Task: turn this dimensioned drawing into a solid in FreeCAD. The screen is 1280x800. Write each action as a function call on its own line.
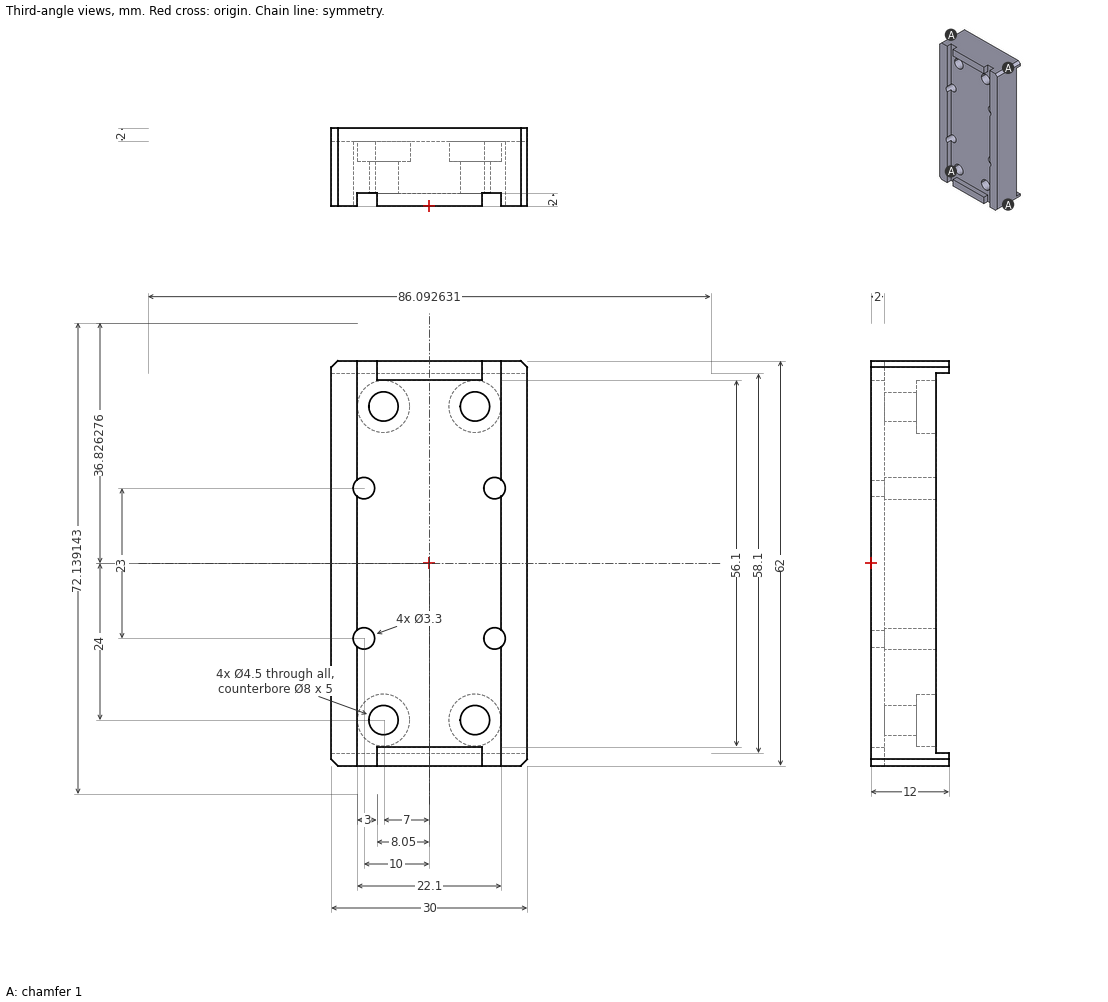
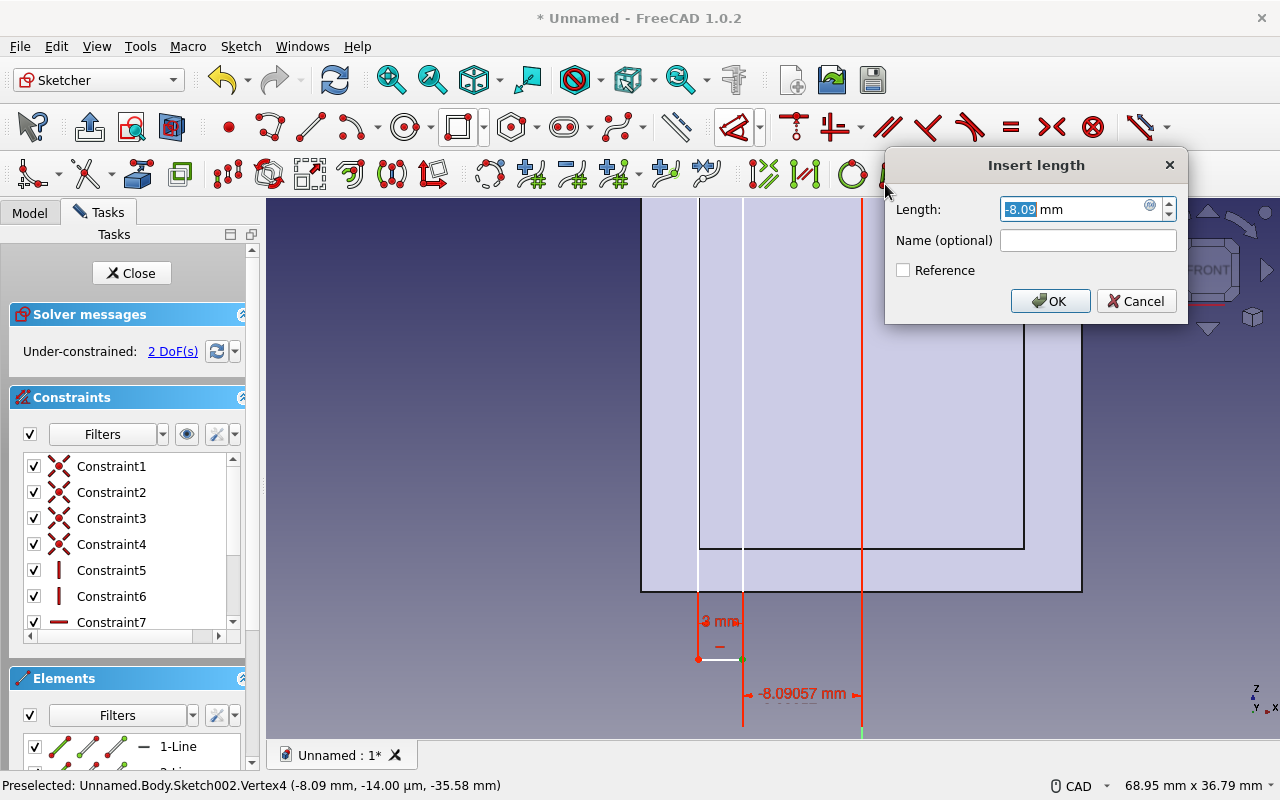
text(-8.05)
key(Return)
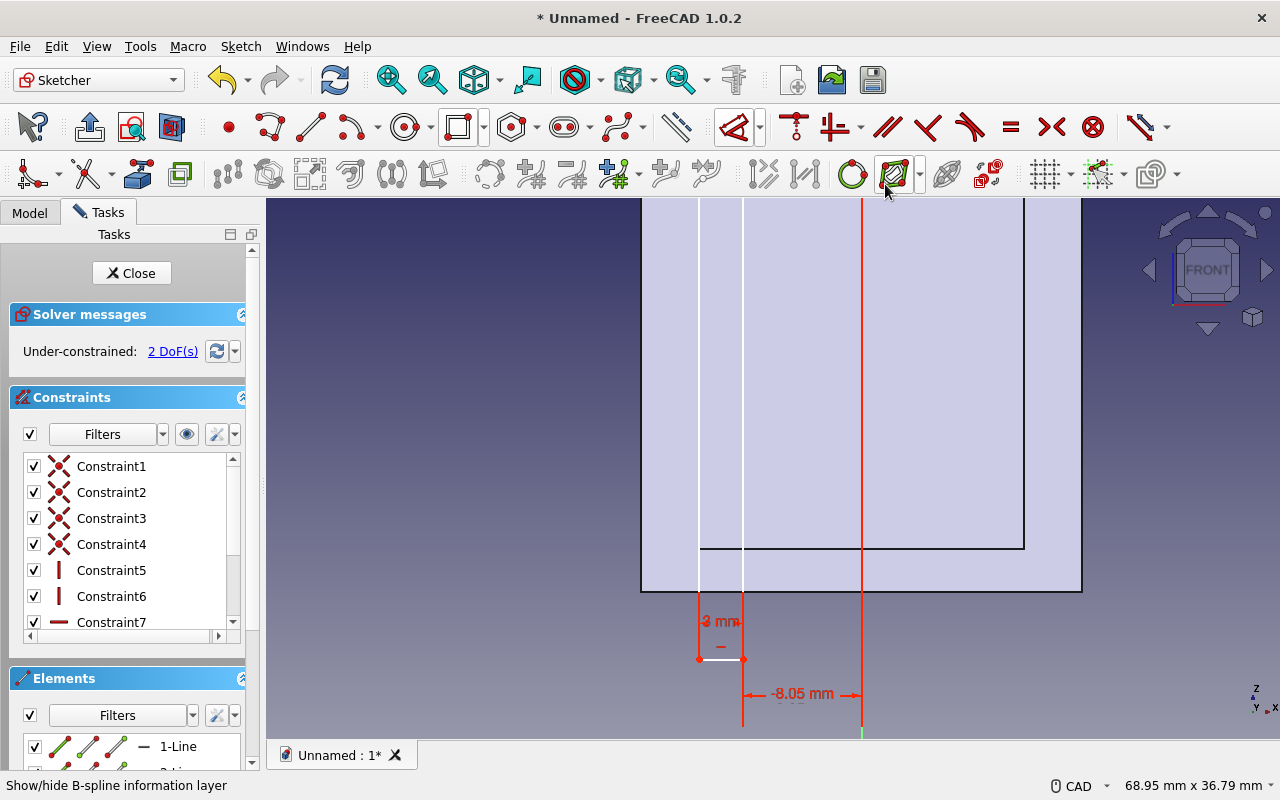
click(699, 341)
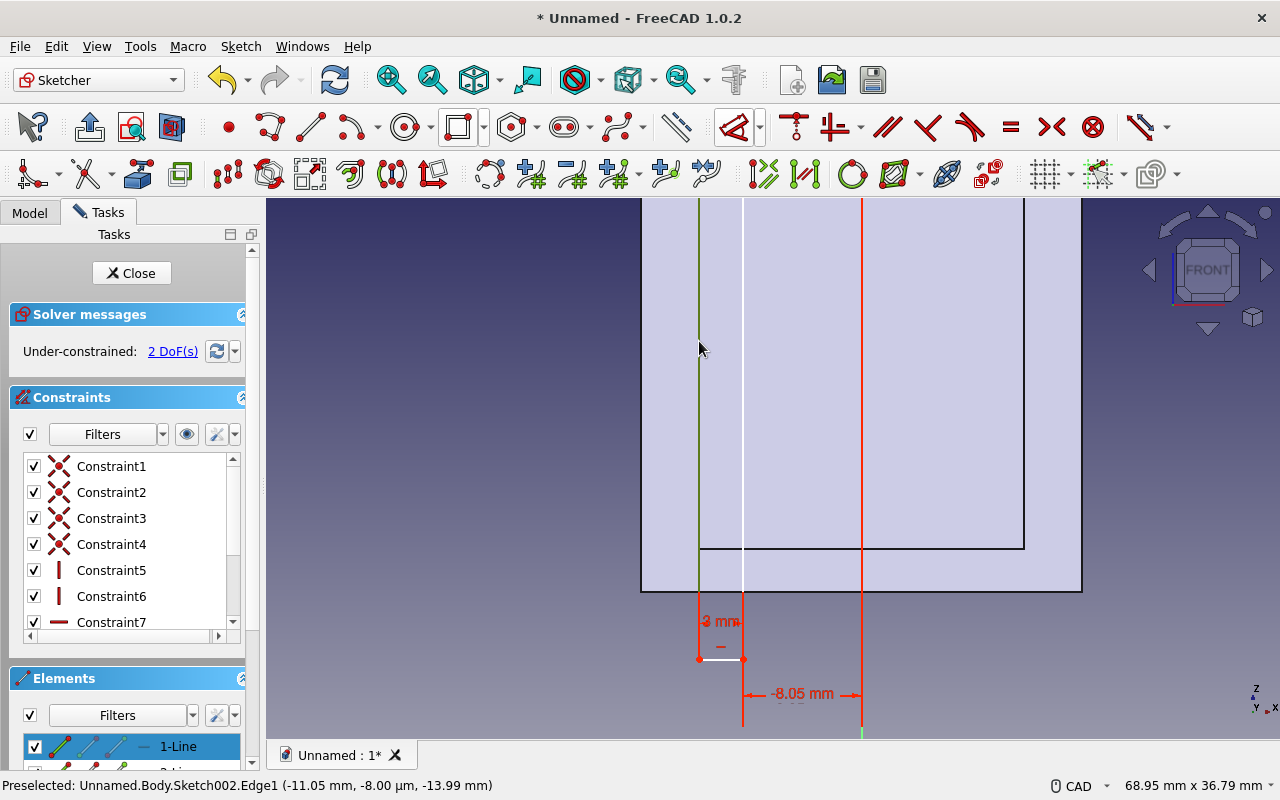
click(760, 128)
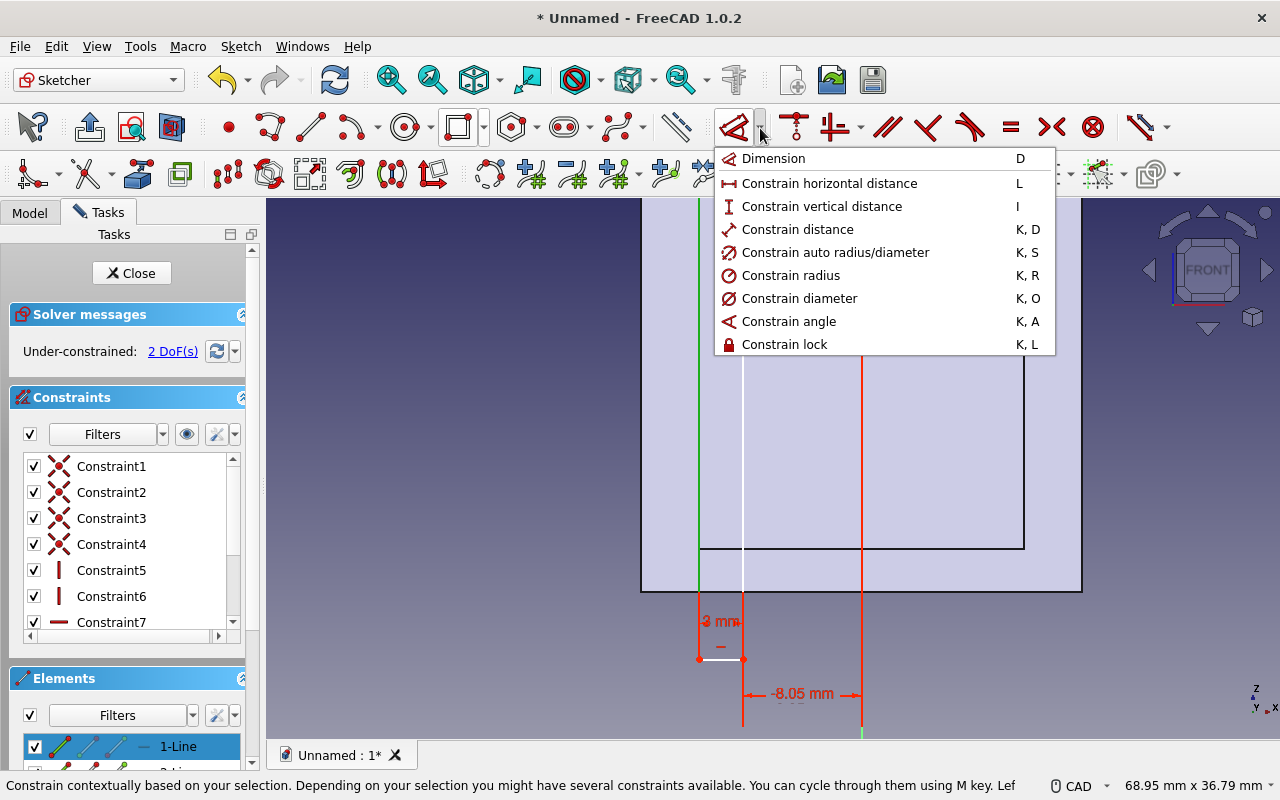
click(885, 206)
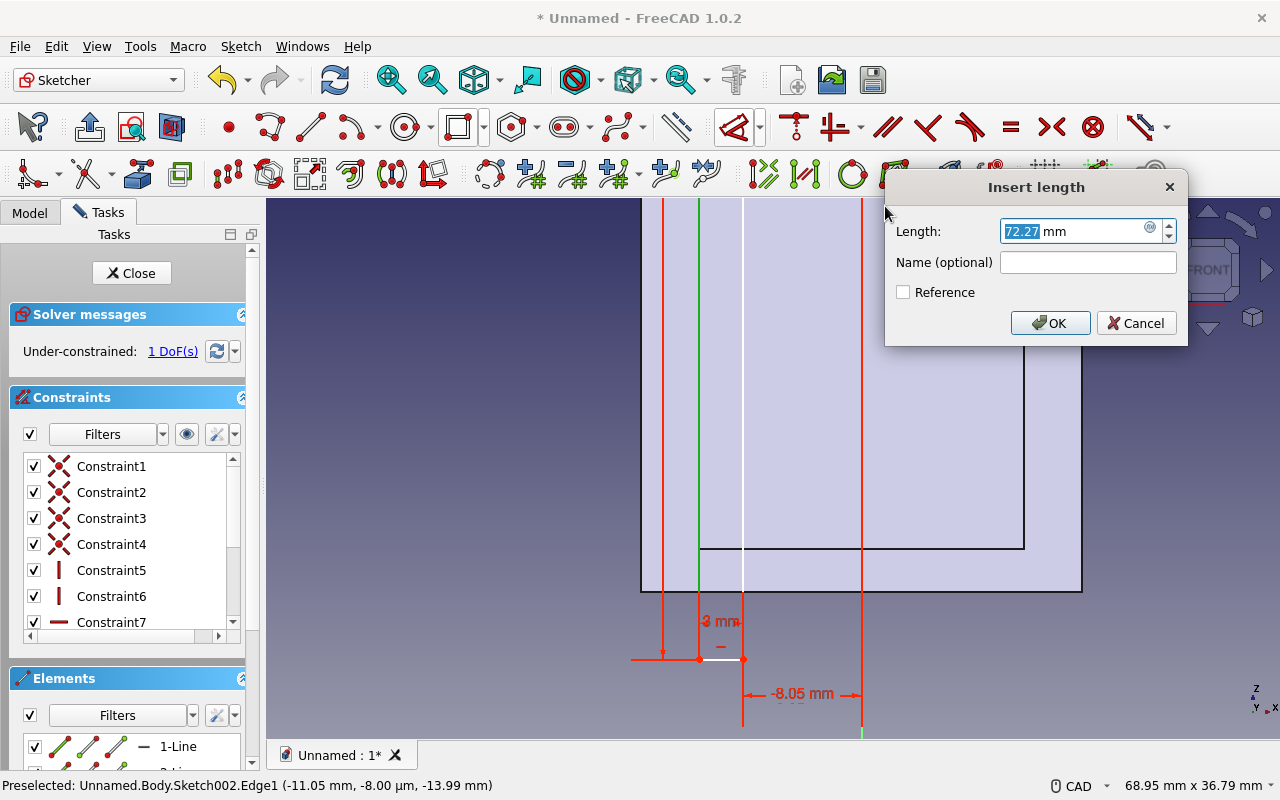
text(72.139143)
key(Return)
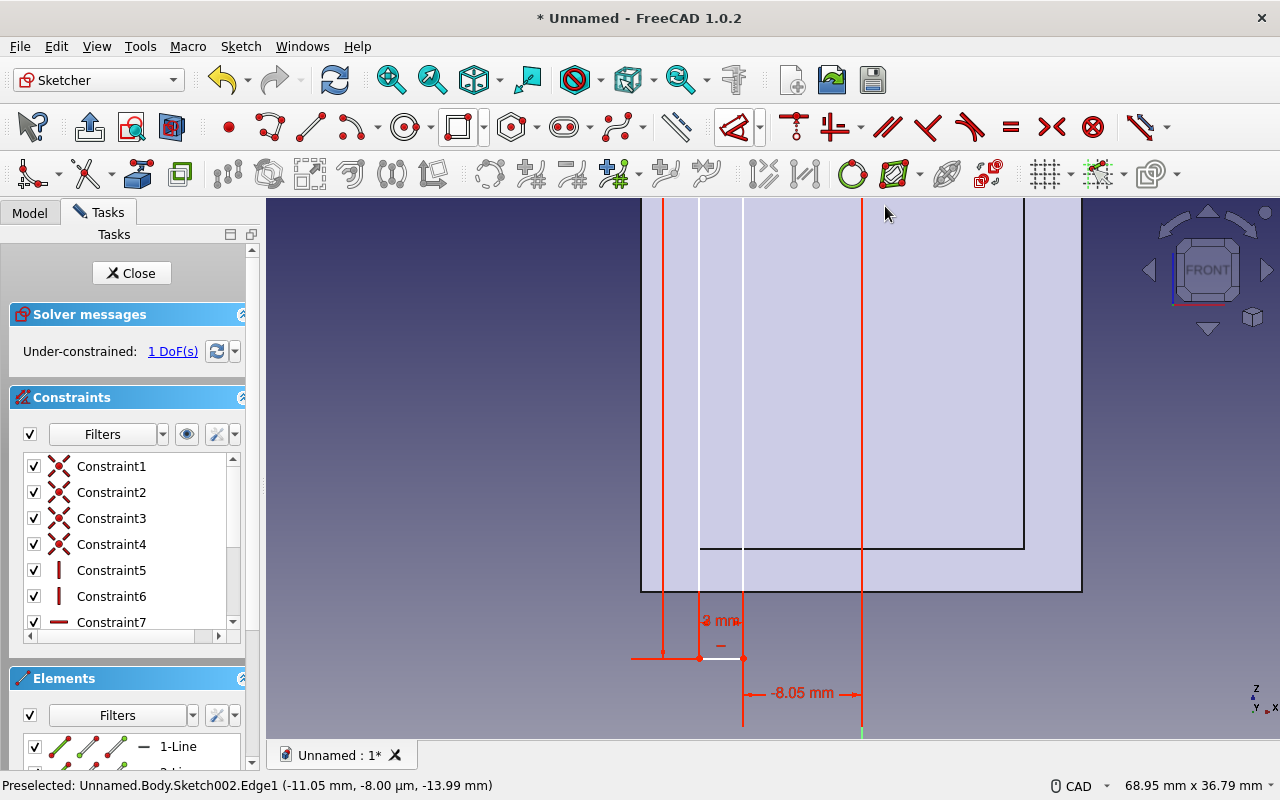
scroll(672, 616, down, 6)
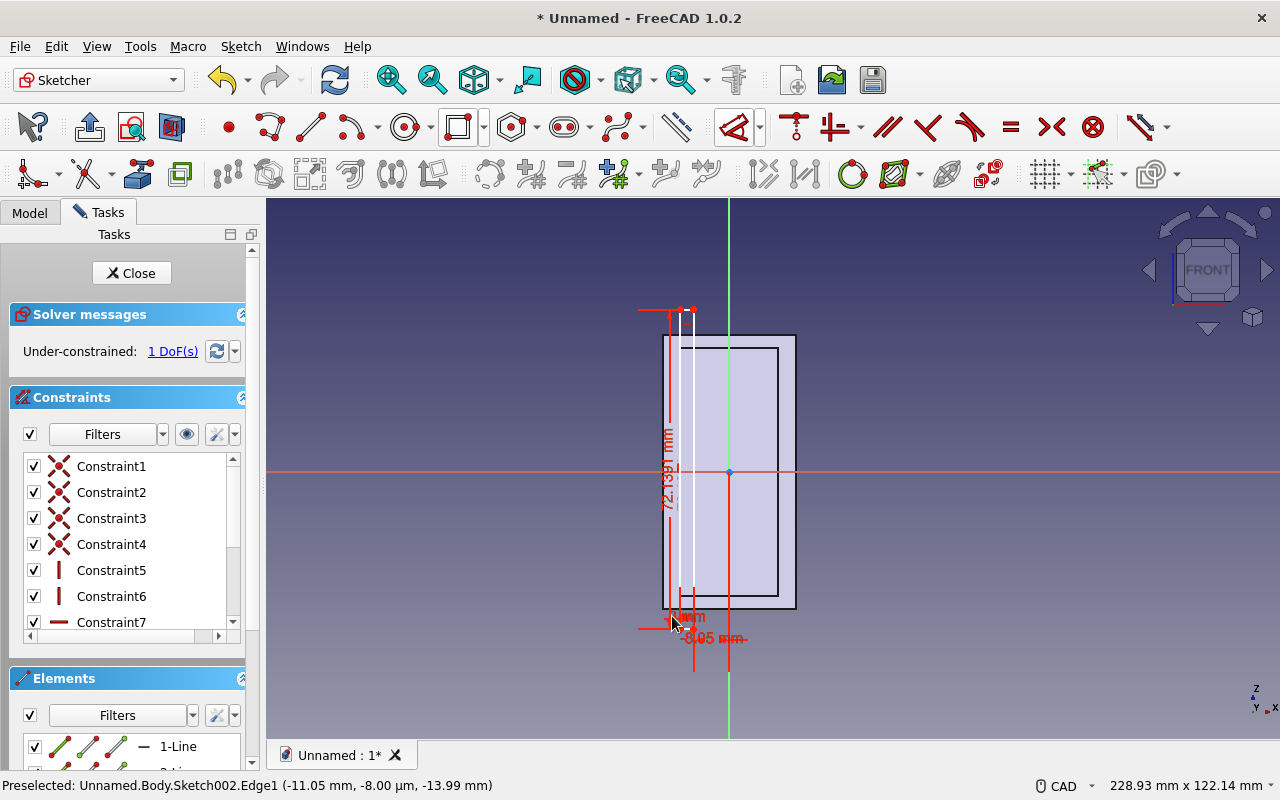
click(680, 310)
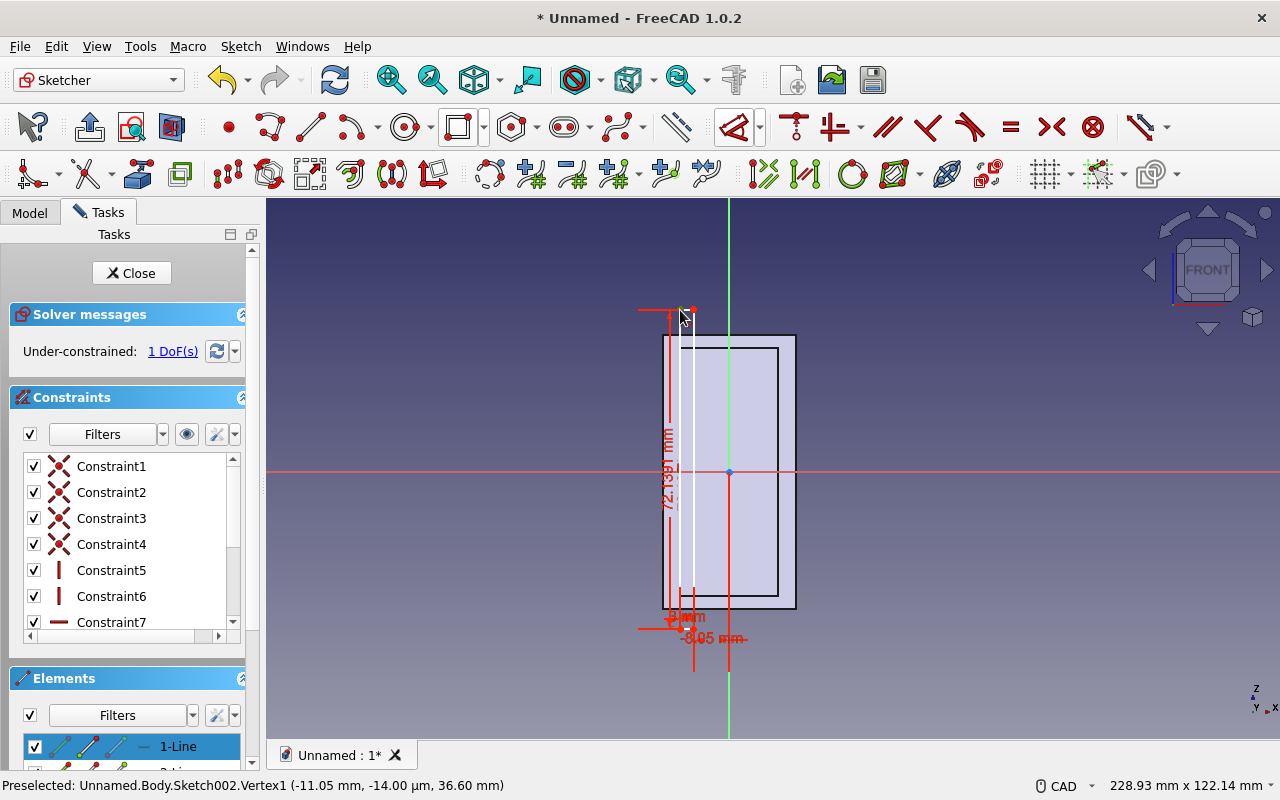
key(i)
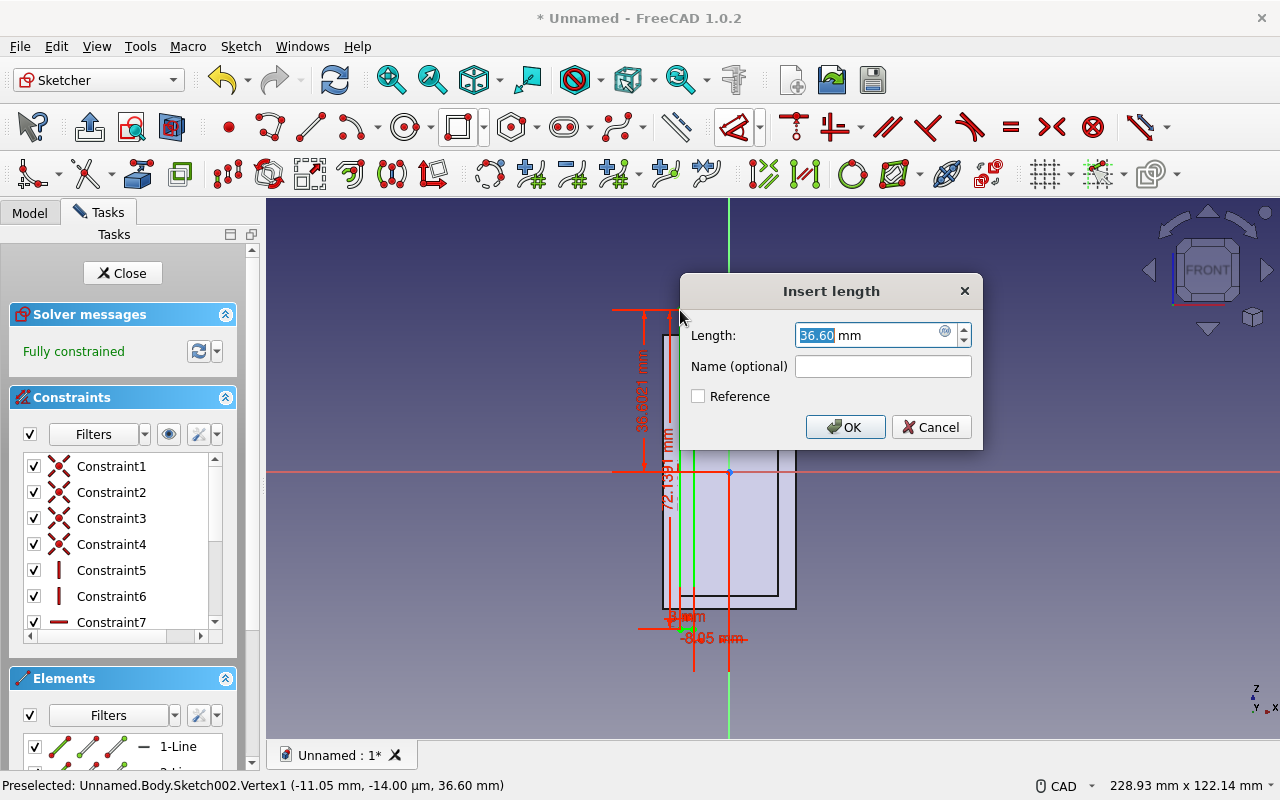
text(36.826276)
key(Return)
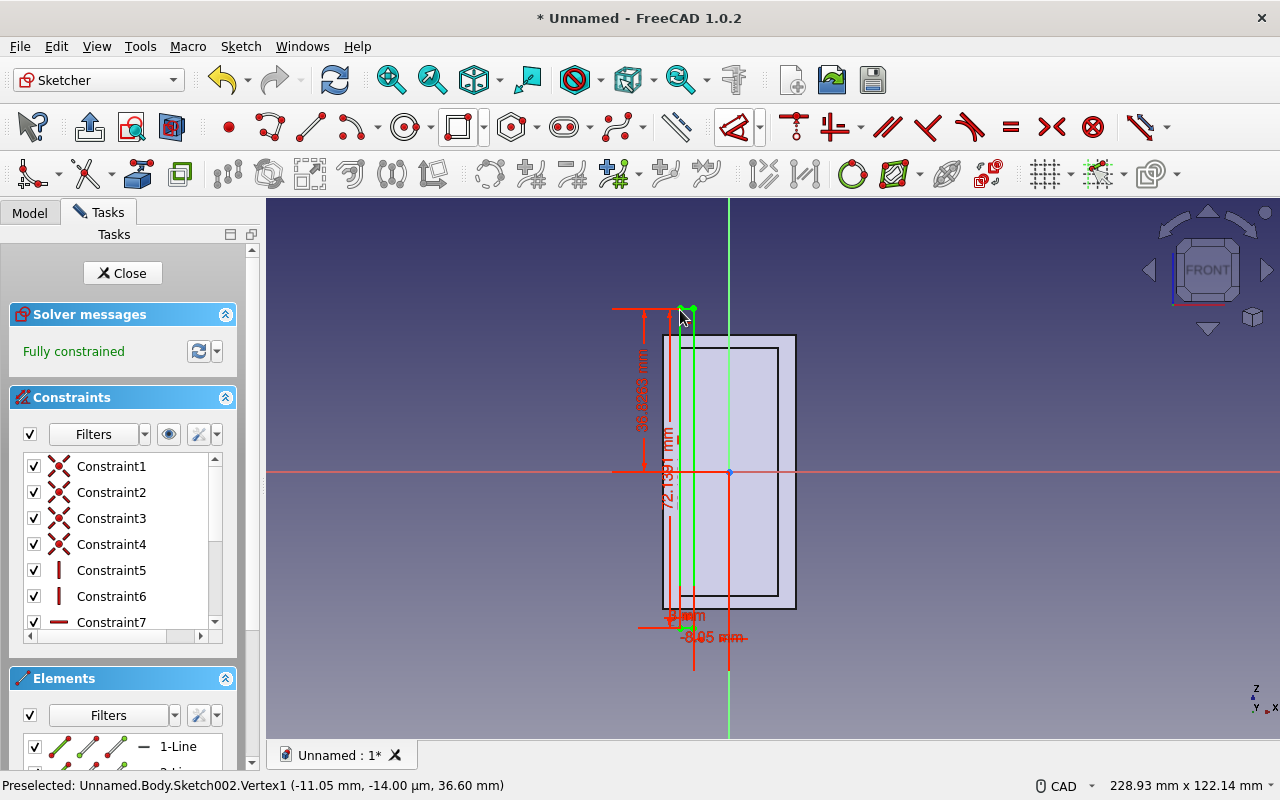
click(123, 273)